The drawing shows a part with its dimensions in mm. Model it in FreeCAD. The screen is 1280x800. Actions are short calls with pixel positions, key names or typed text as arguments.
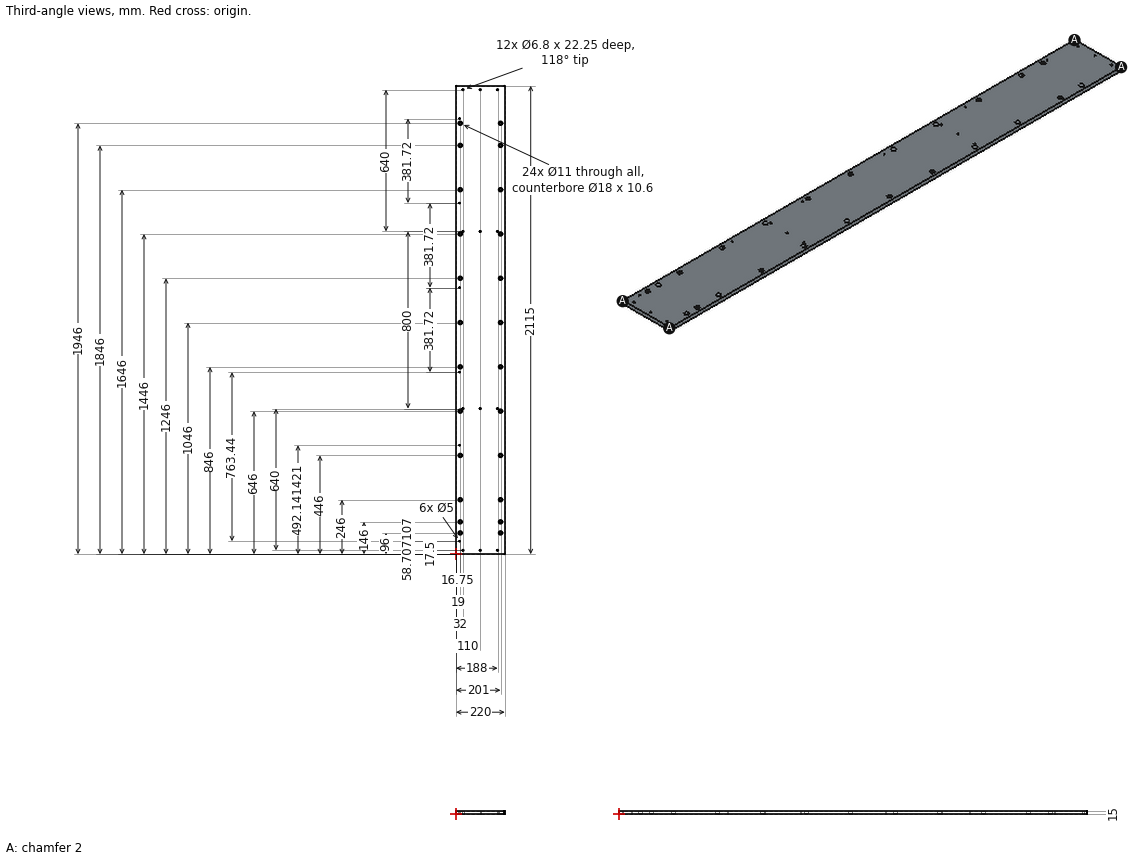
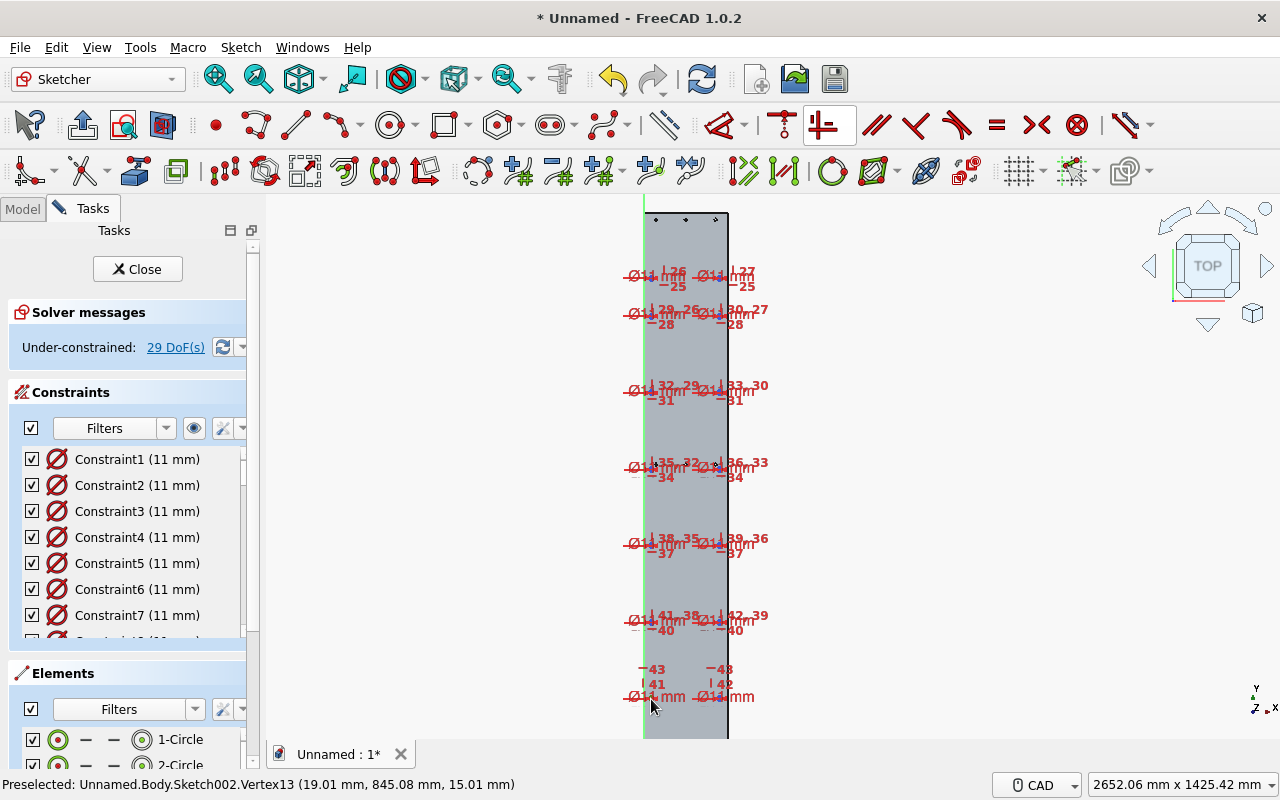
scroll(722, 318, down, 4)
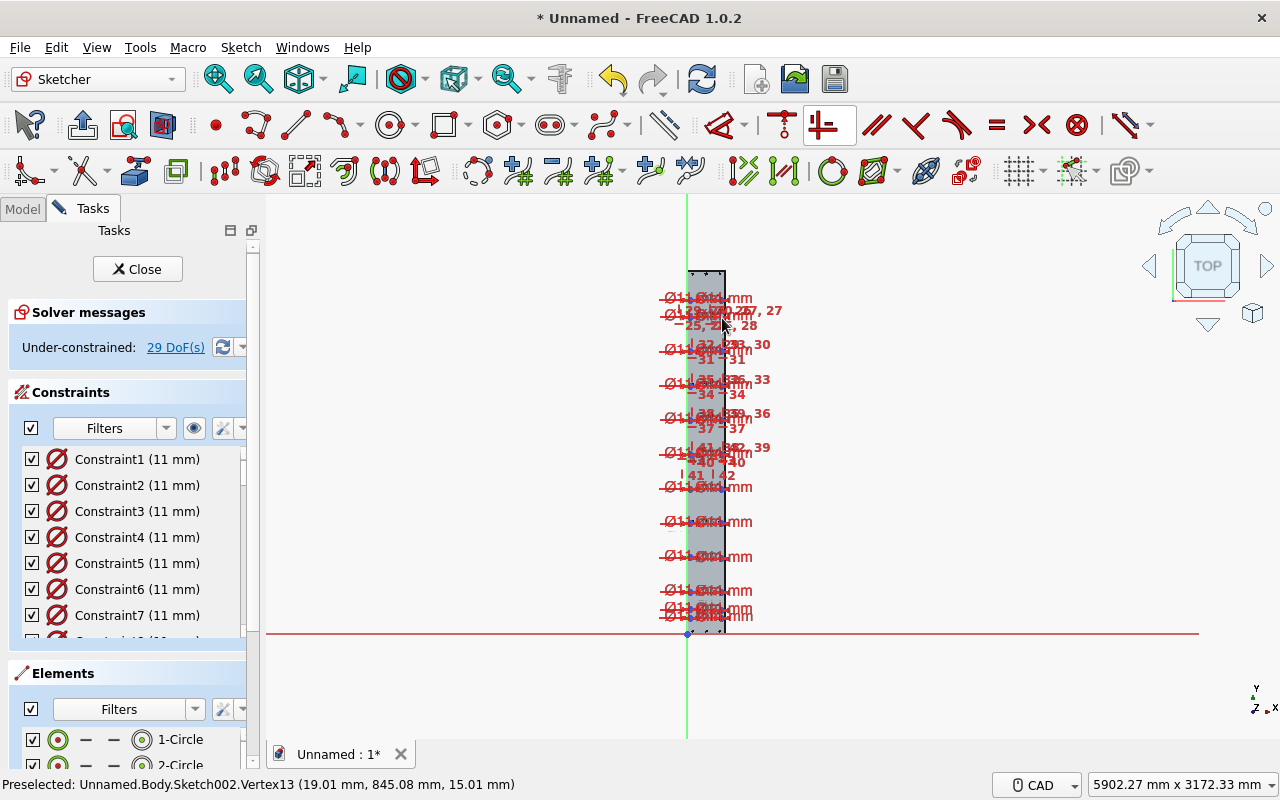
click(690, 524)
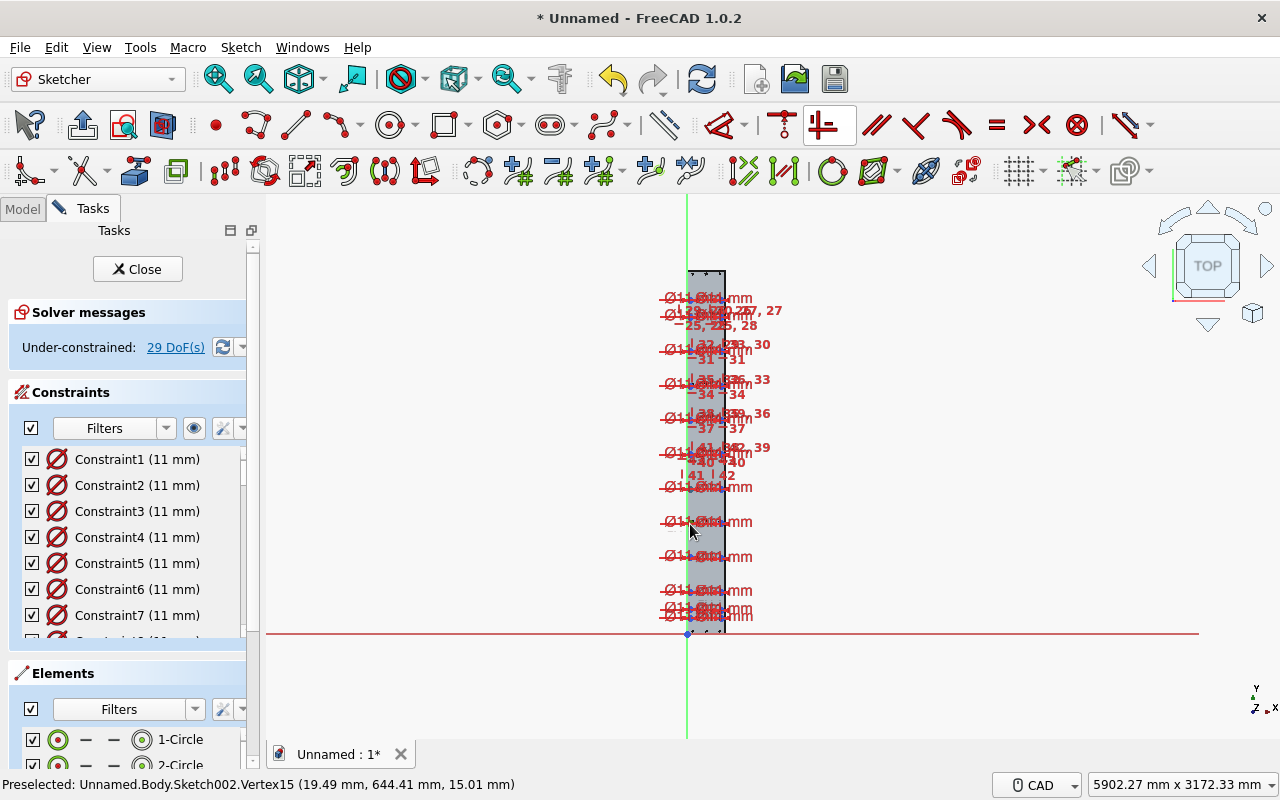
click(850, 126)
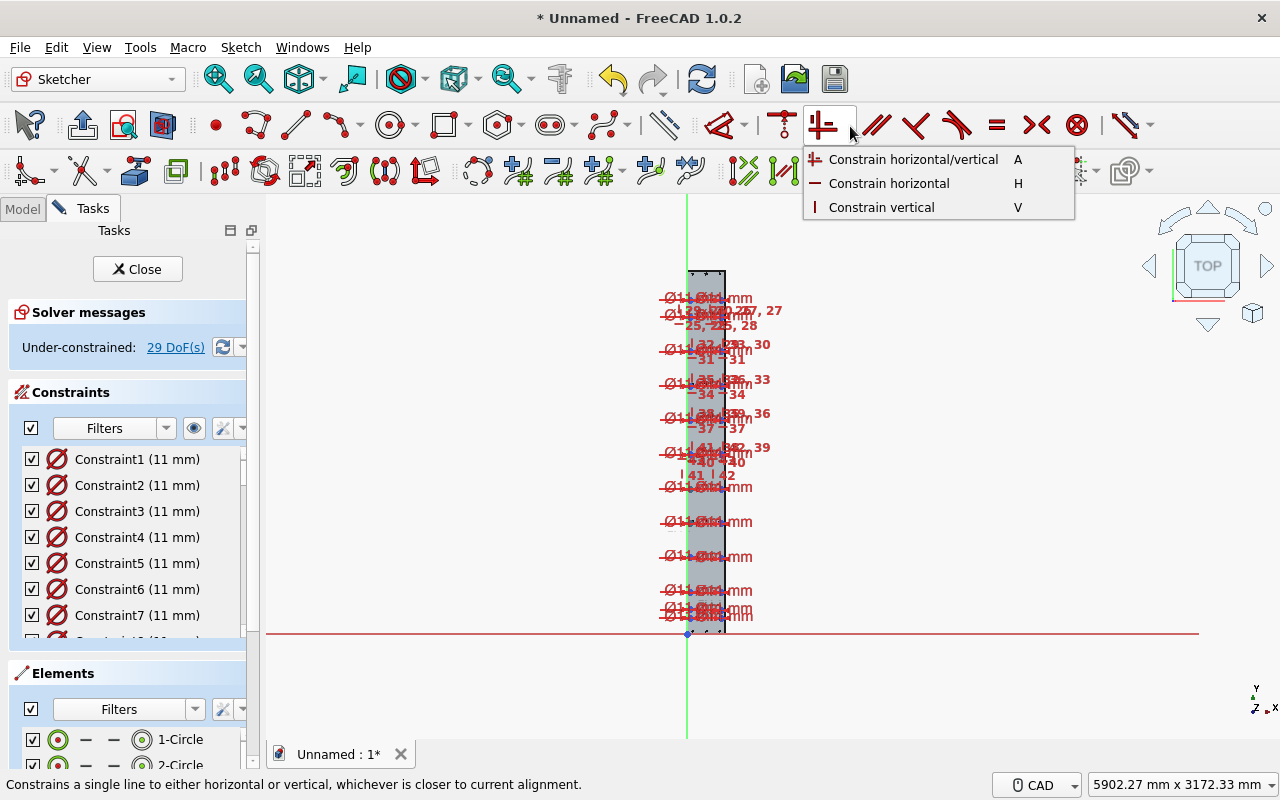
click(939, 207)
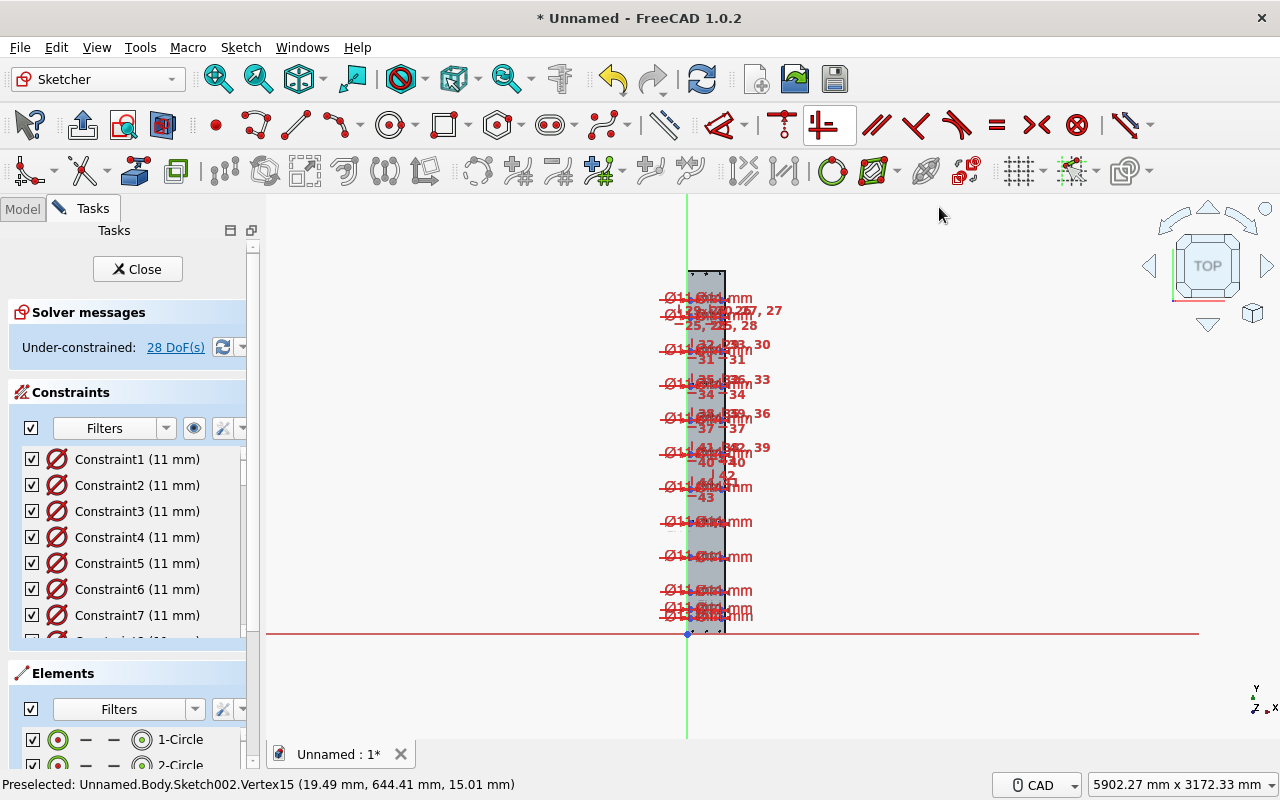
click(721, 489)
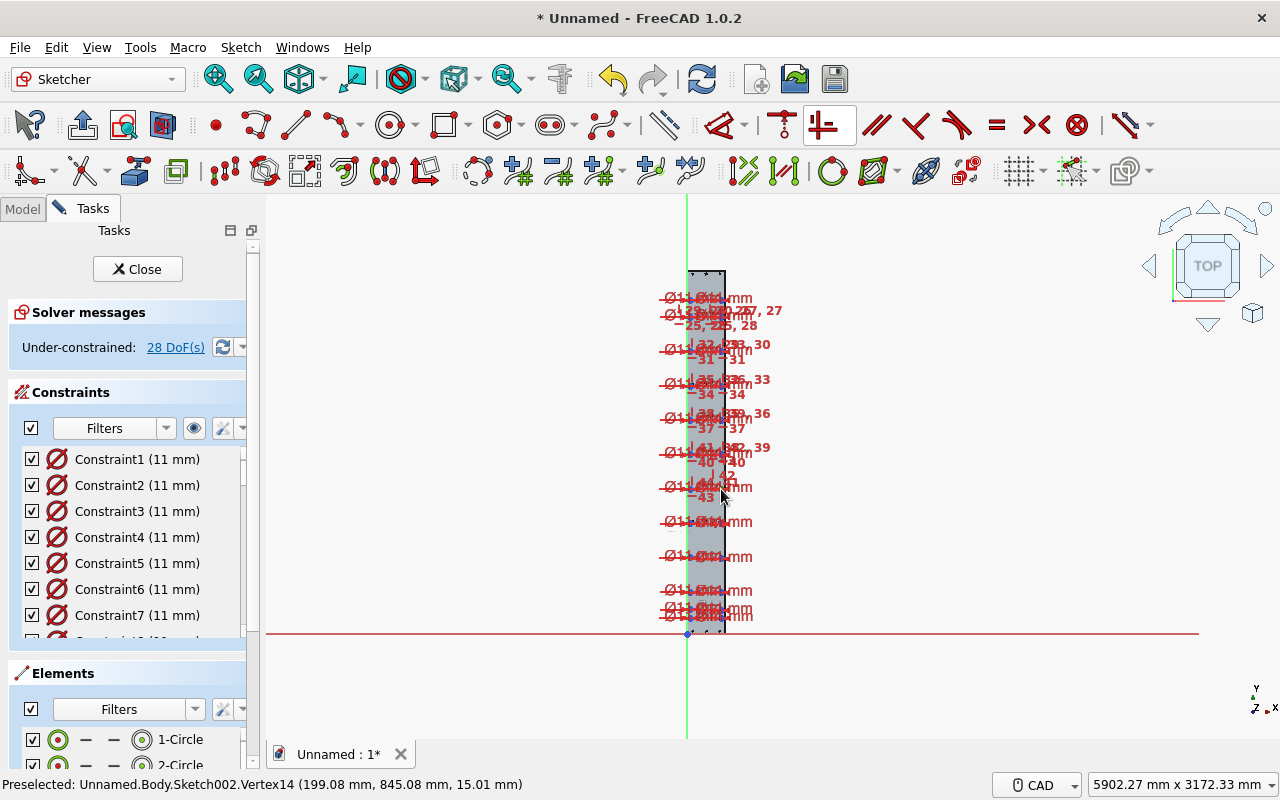
scroll(721, 524, up, 4)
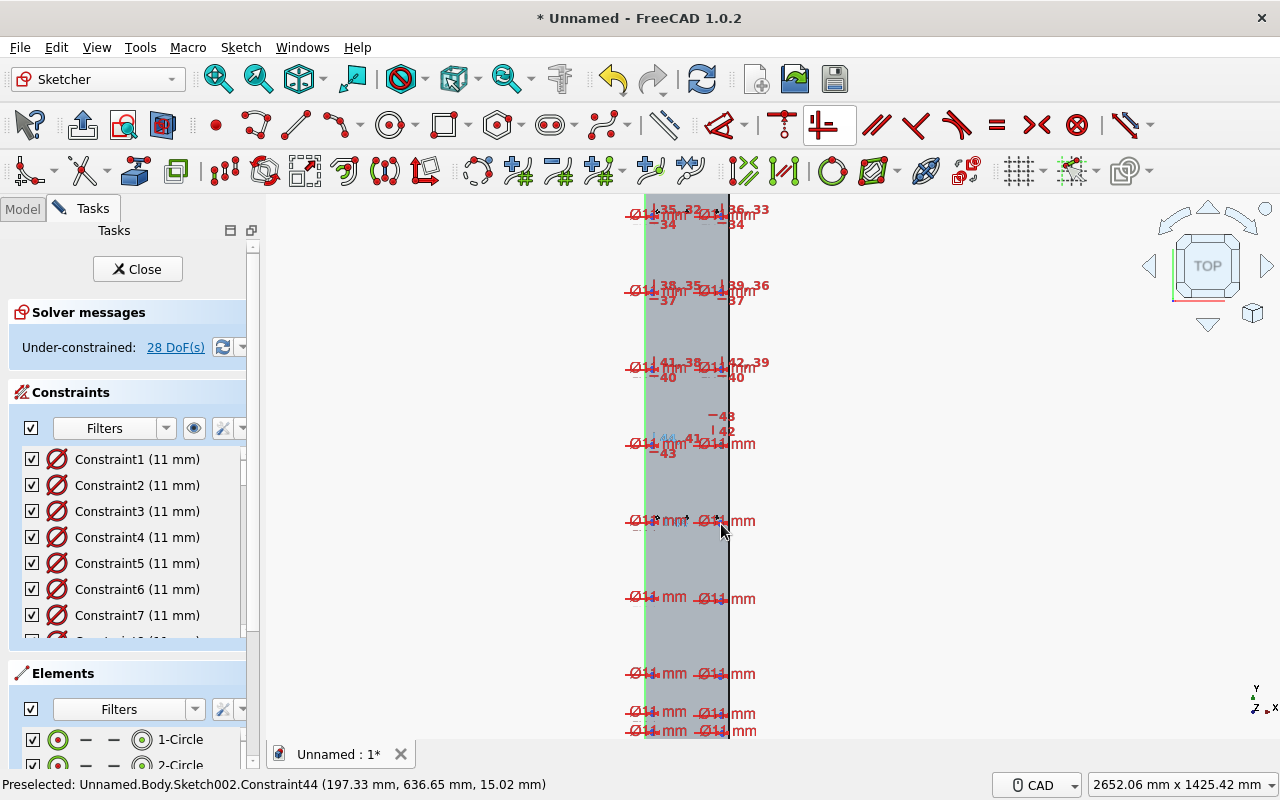
click(721, 523)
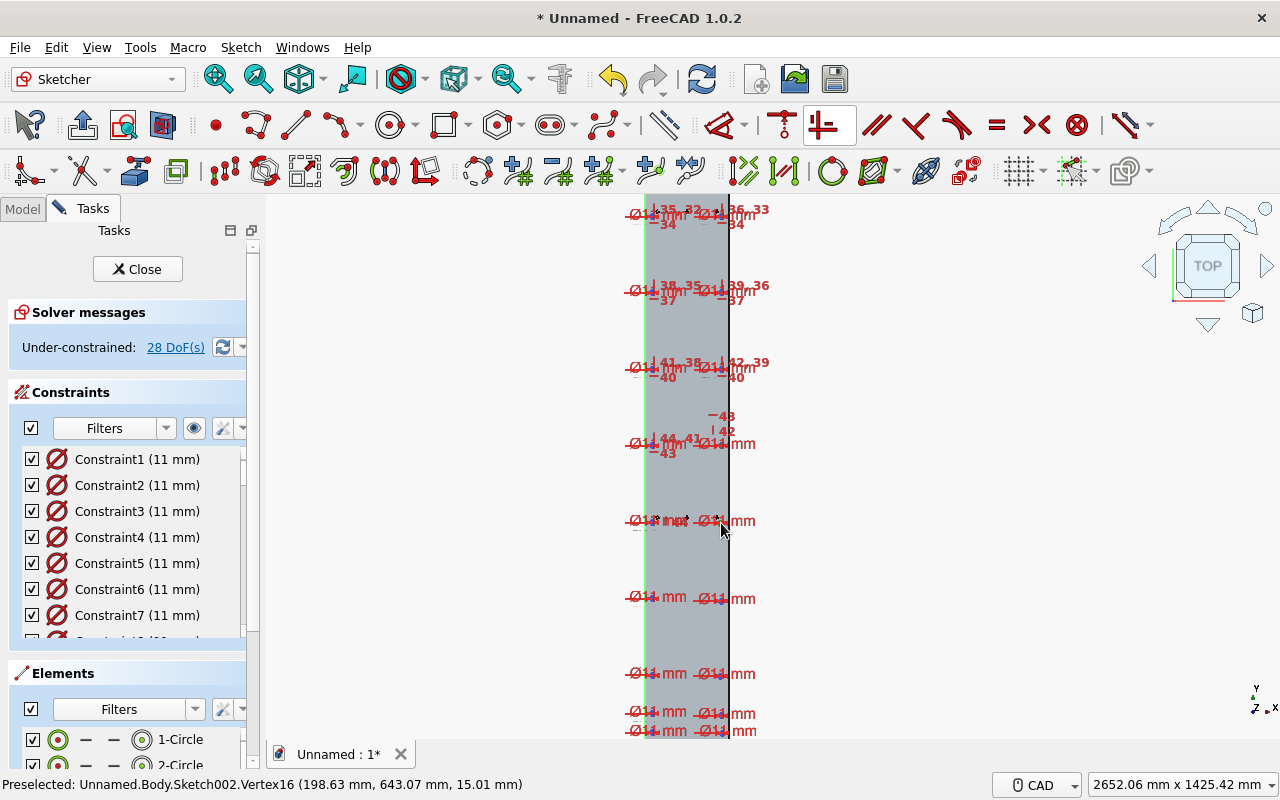
click(850, 126)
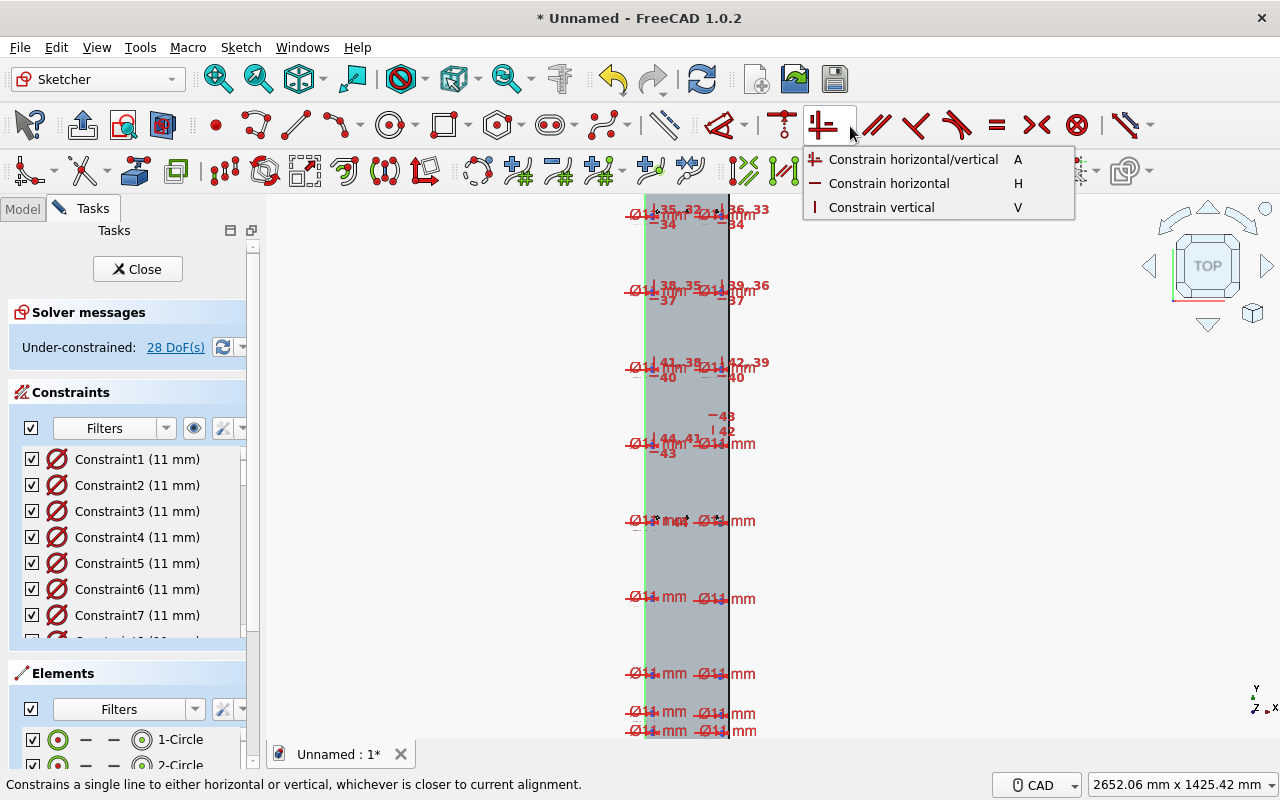
click(939, 207)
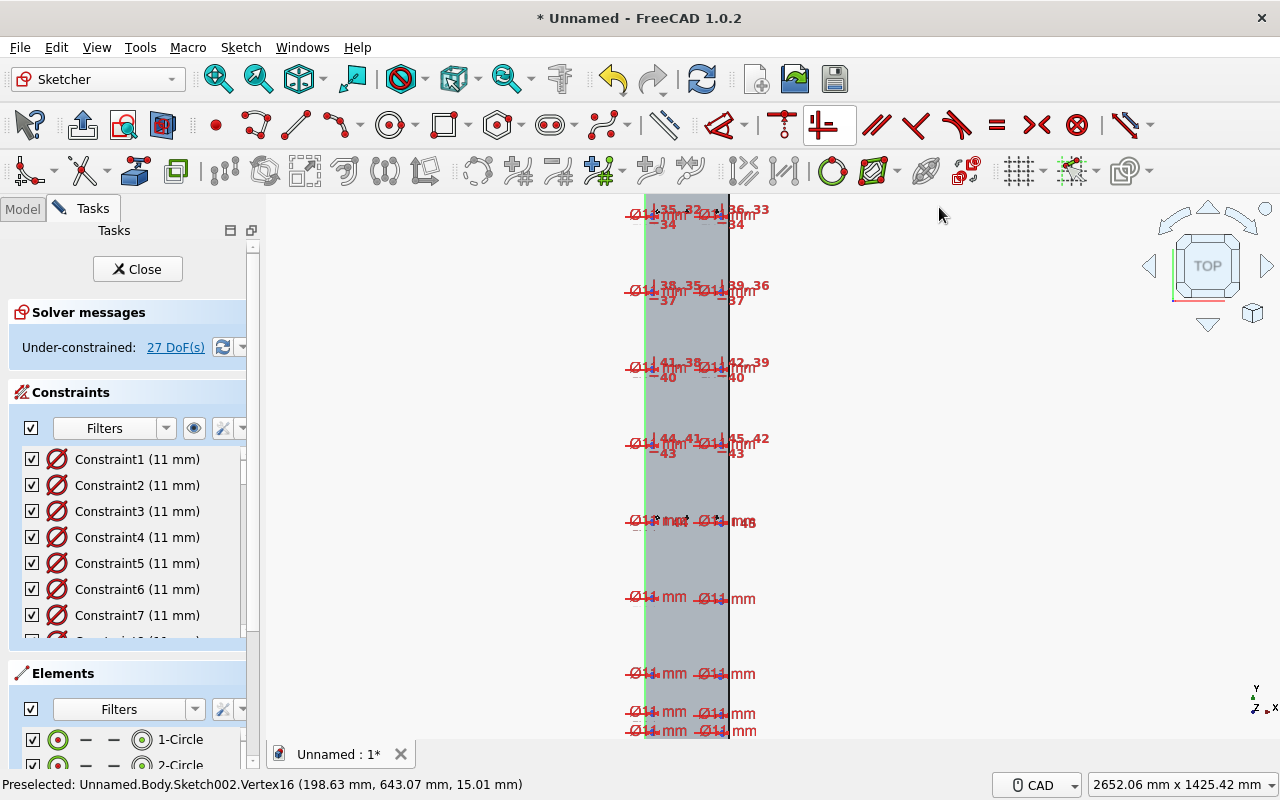
click(652, 523)